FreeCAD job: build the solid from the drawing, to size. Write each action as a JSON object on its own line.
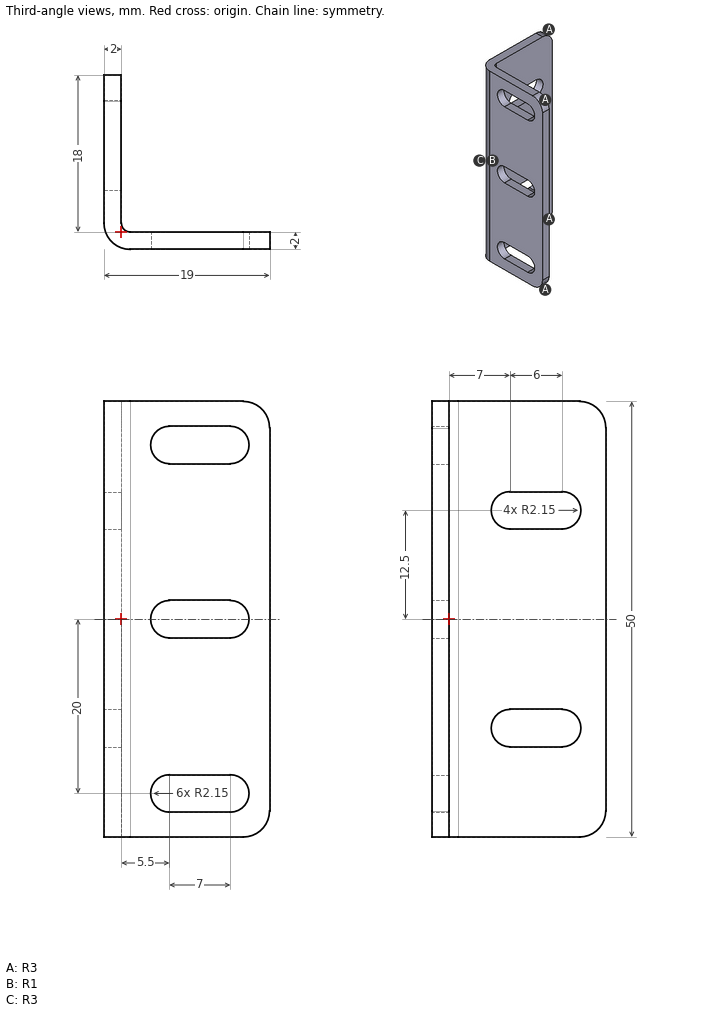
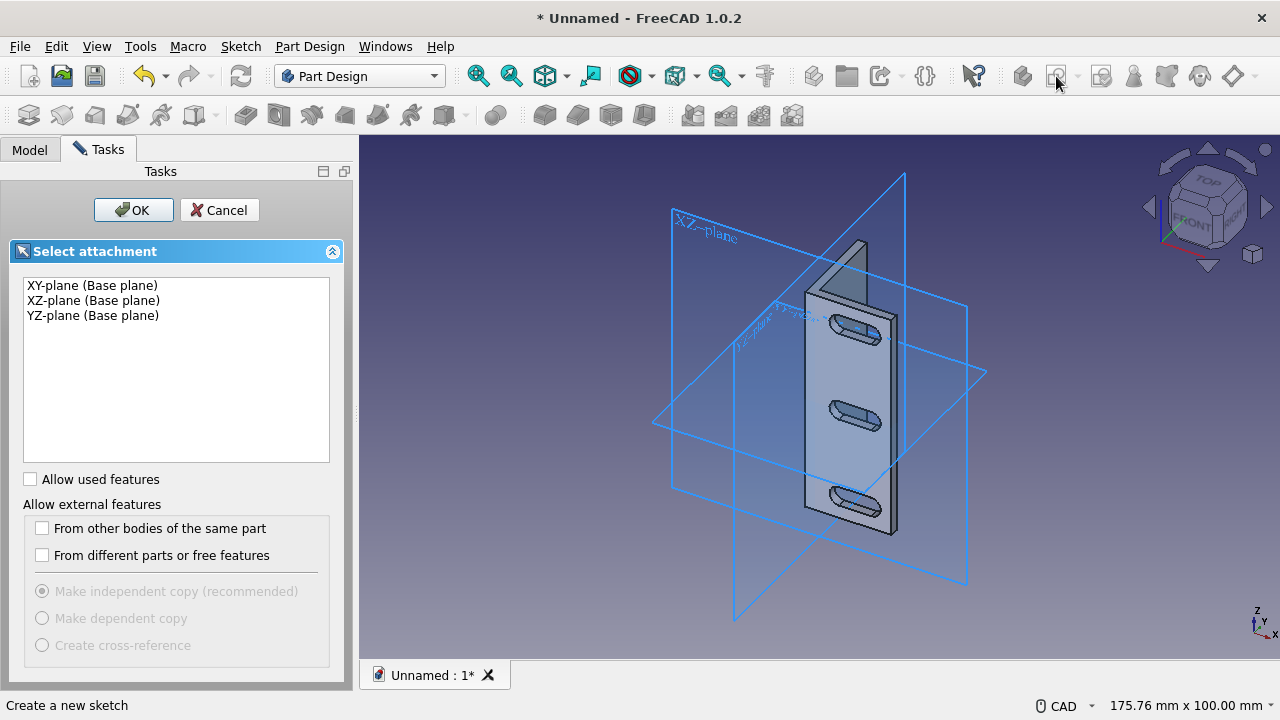
{"action": "left_click", "coordinate": [84, 316]}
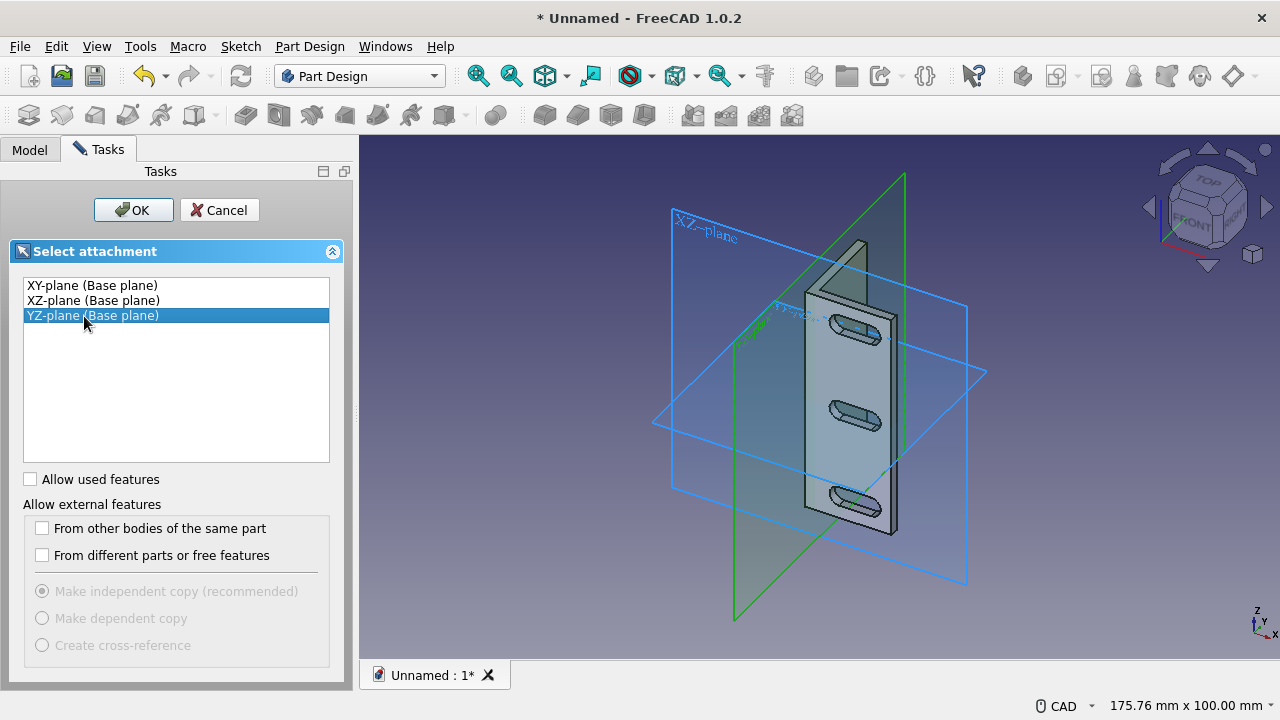
{"action": "left_click", "coordinate": [134, 210]}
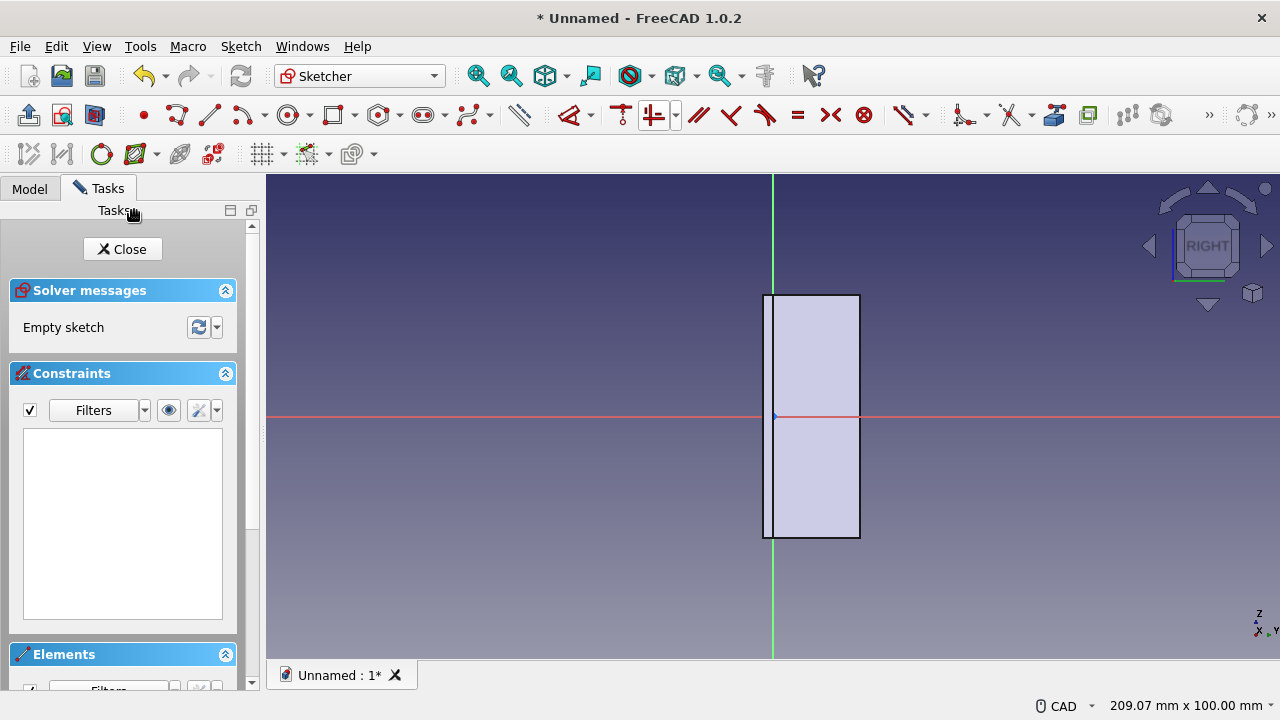
{"action": "left_click", "coordinate": [95, 116]}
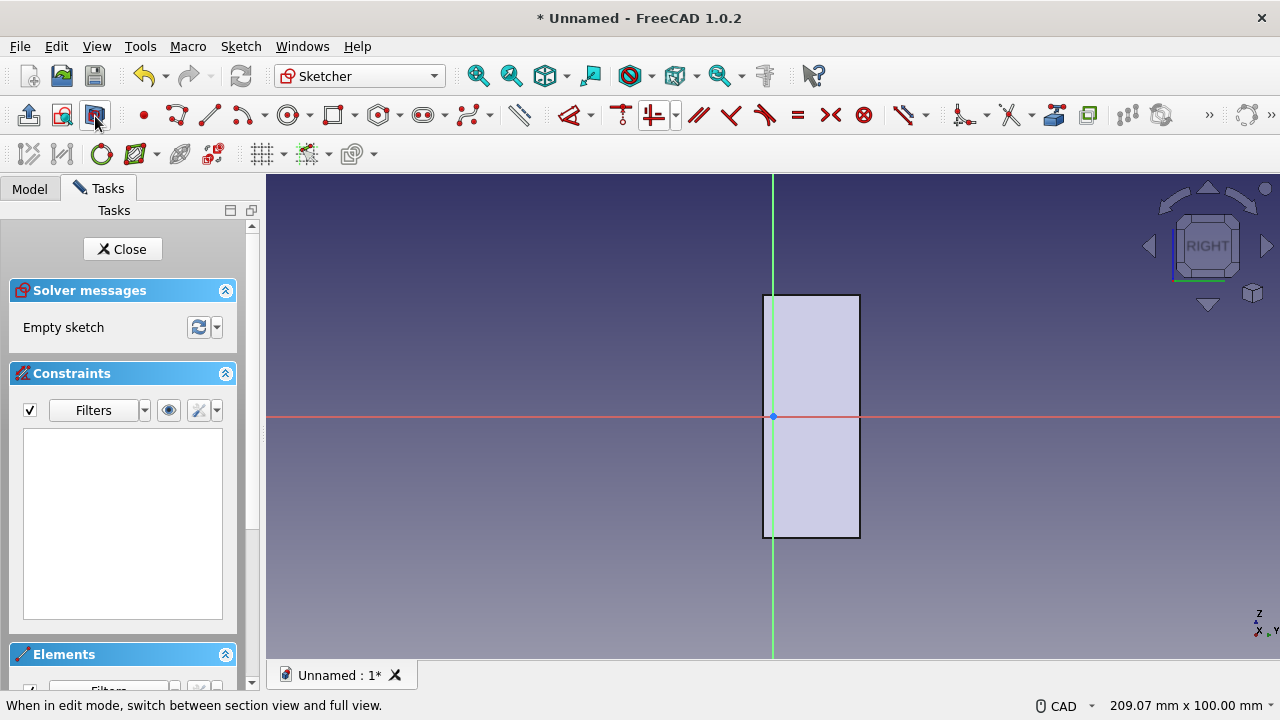
{"action": "scroll", "coordinate": [896, 416], "scroll_direction": "up", "scroll_amount": 4}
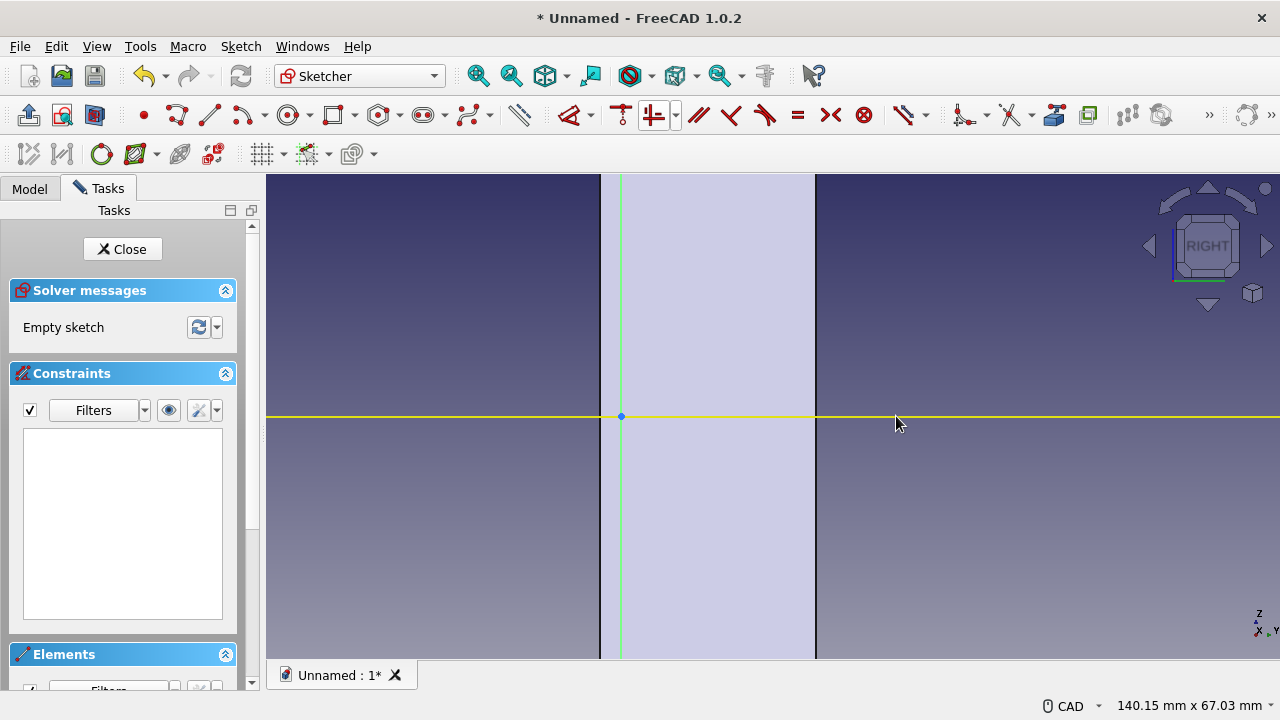
{"action": "left_click", "coordinate": [422, 116]}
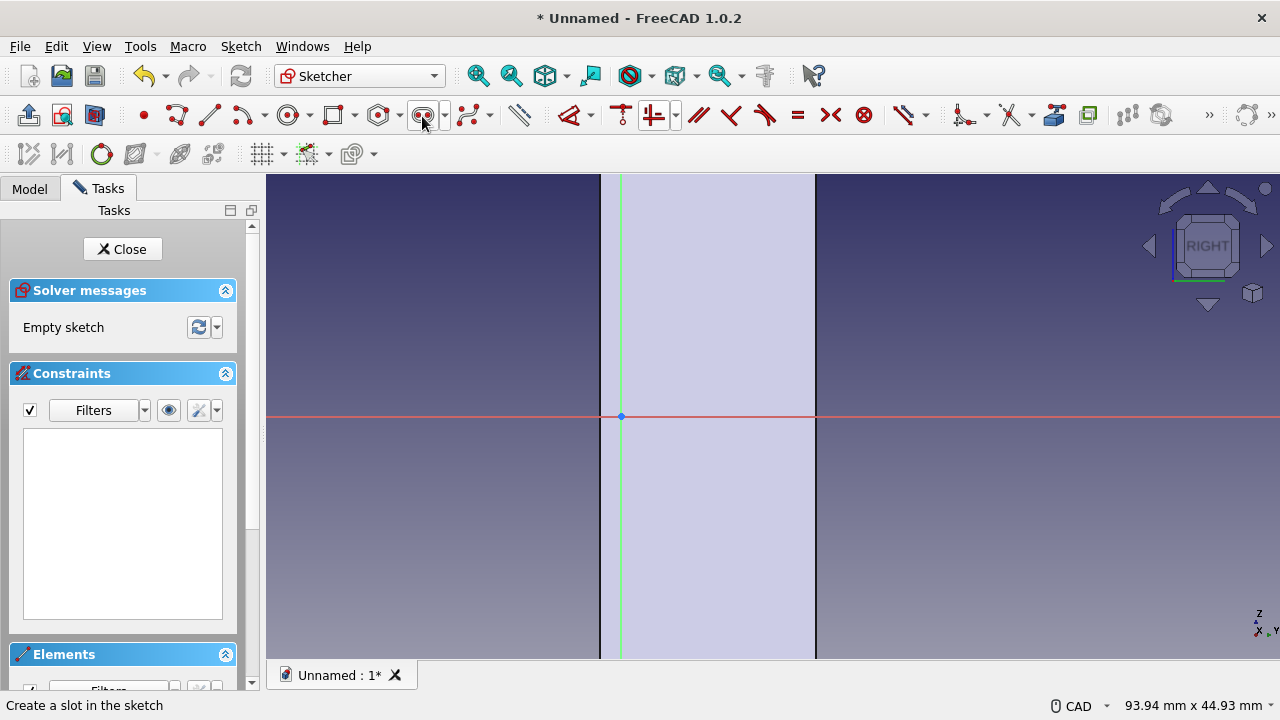
{"action": "left_click", "coordinate": [697, 282]}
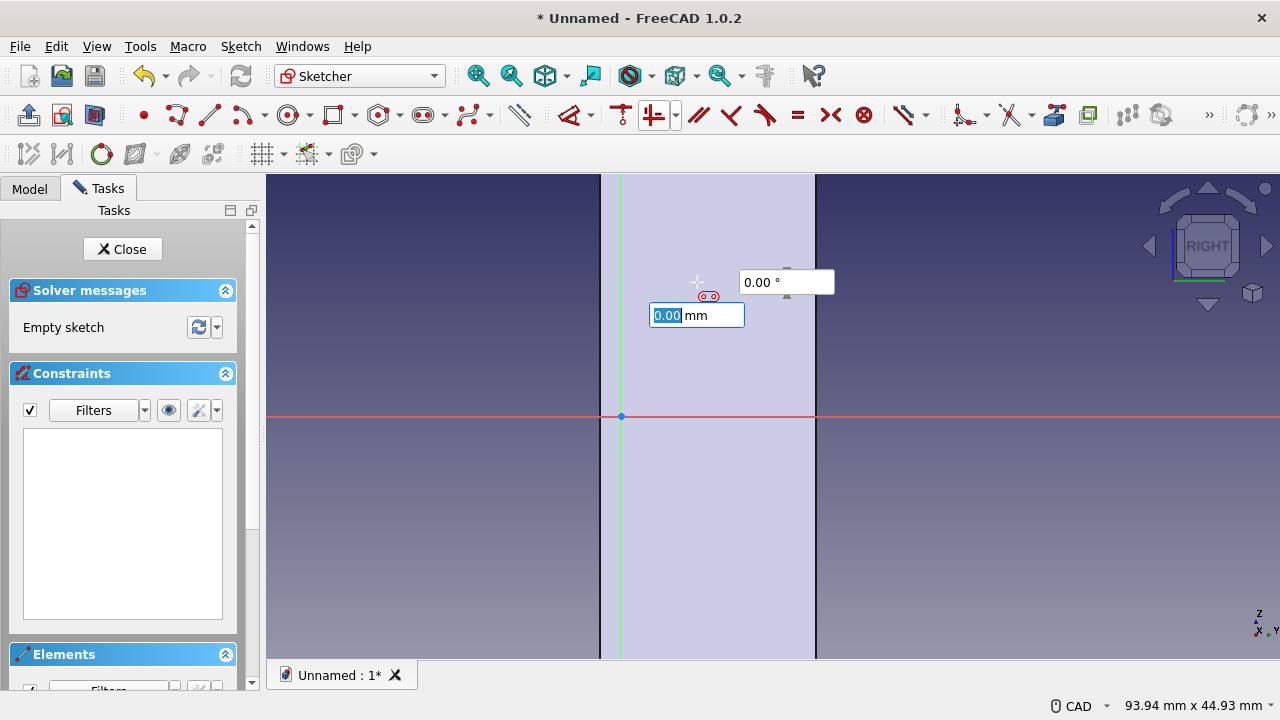
{"action": "left_click", "coordinate": [762, 282]}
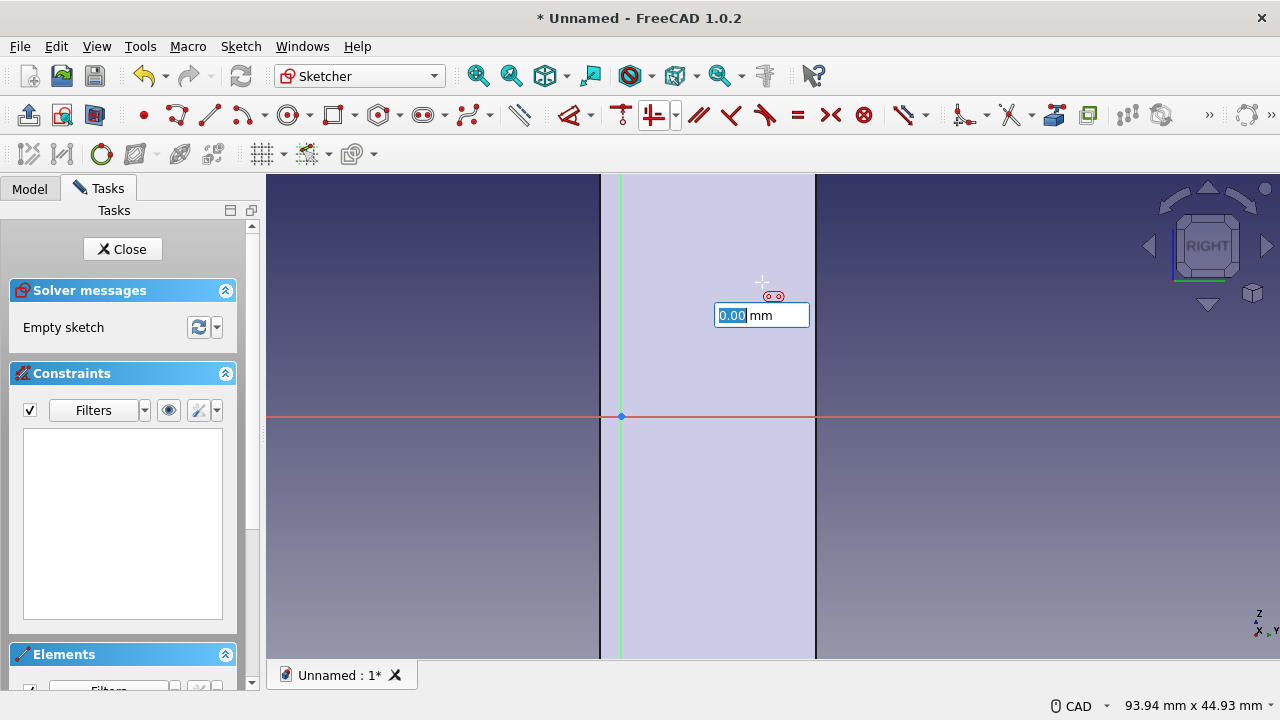
{"action": "left_click", "coordinate": [729, 305]}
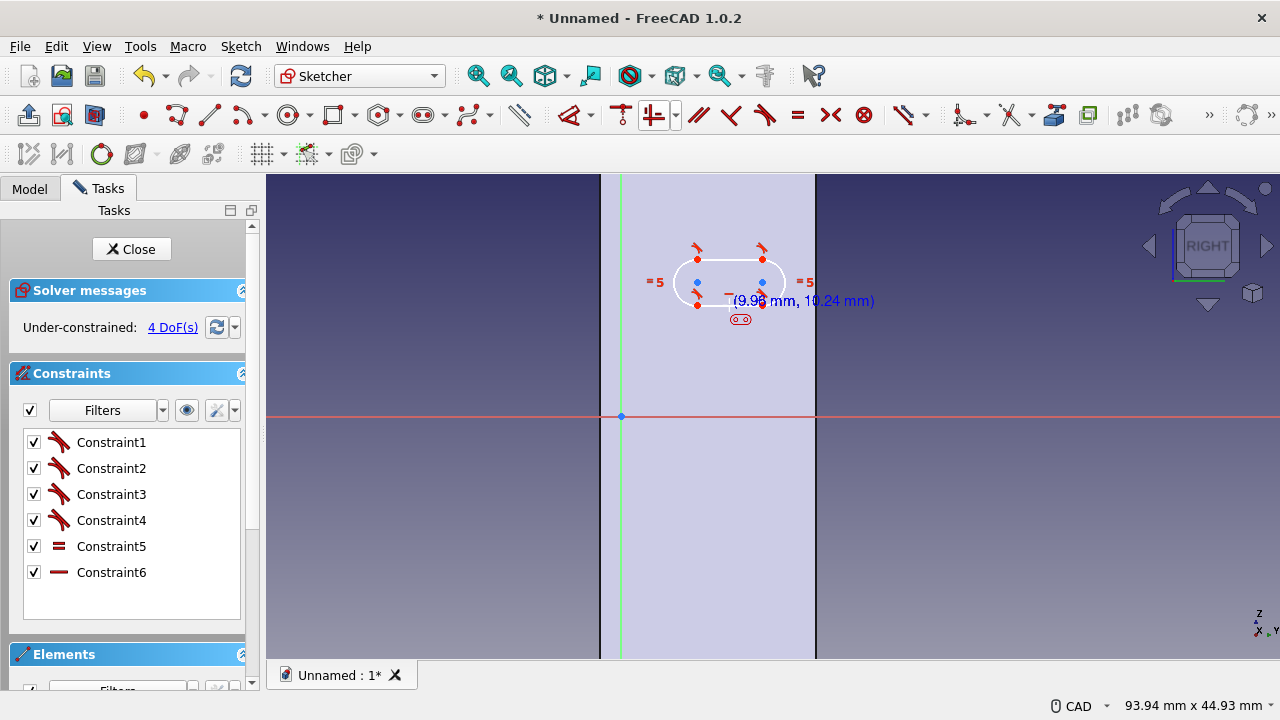
{"action": "left_click", "coordinate": [697, 551]}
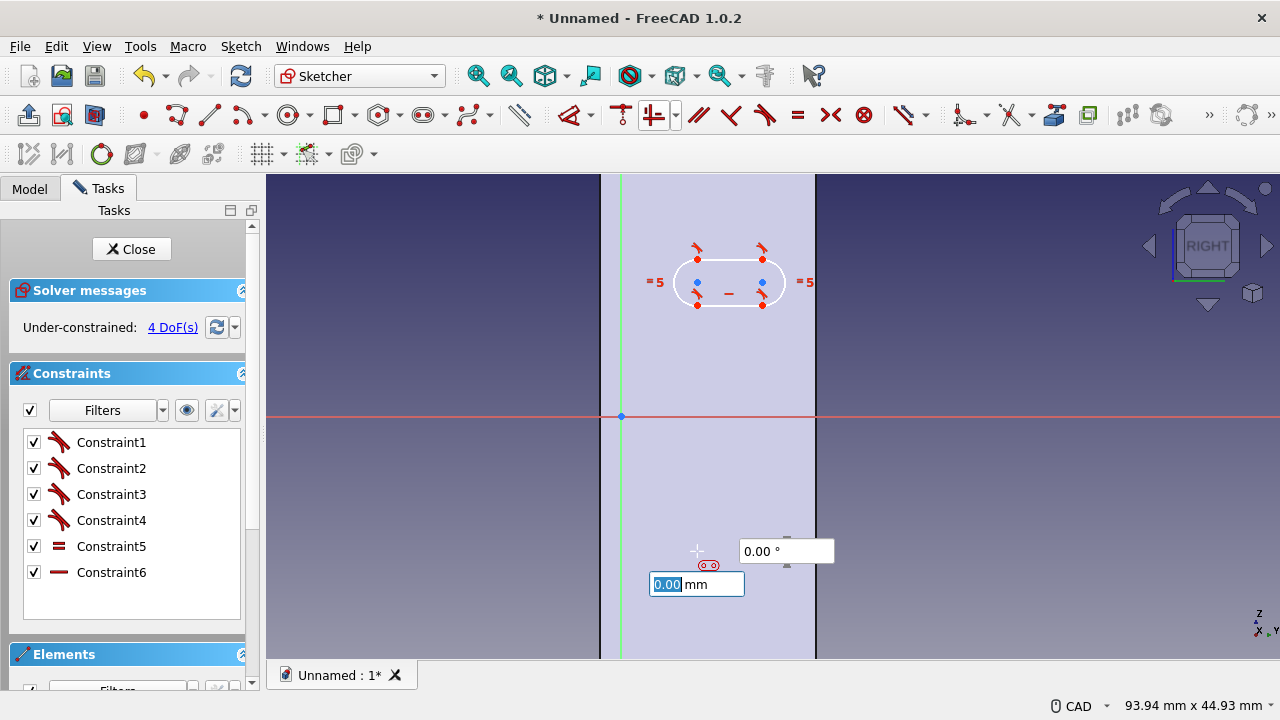
{"action": "left_click", "coordinate": [762, 551]}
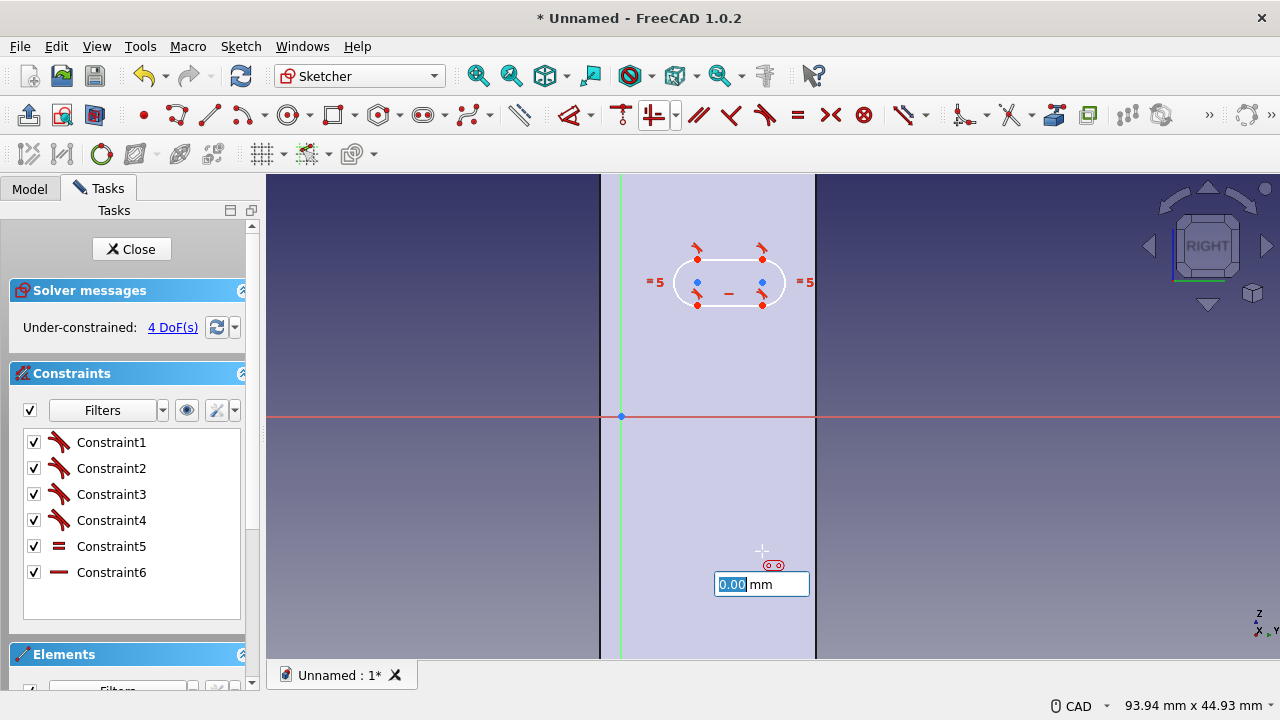
{"action": "left_click", "coordinate": [729, 528]}
{"action": "key", "text": "Escape"}